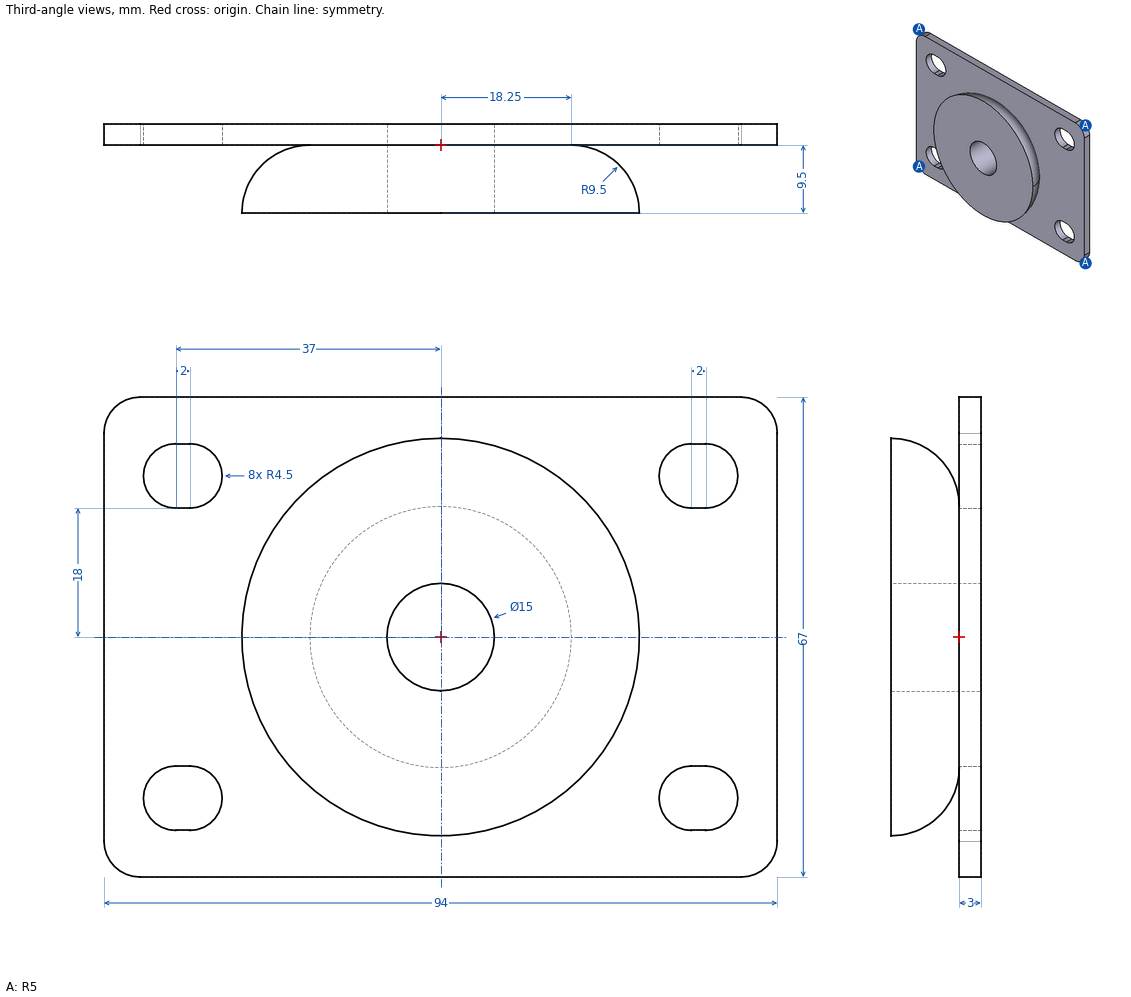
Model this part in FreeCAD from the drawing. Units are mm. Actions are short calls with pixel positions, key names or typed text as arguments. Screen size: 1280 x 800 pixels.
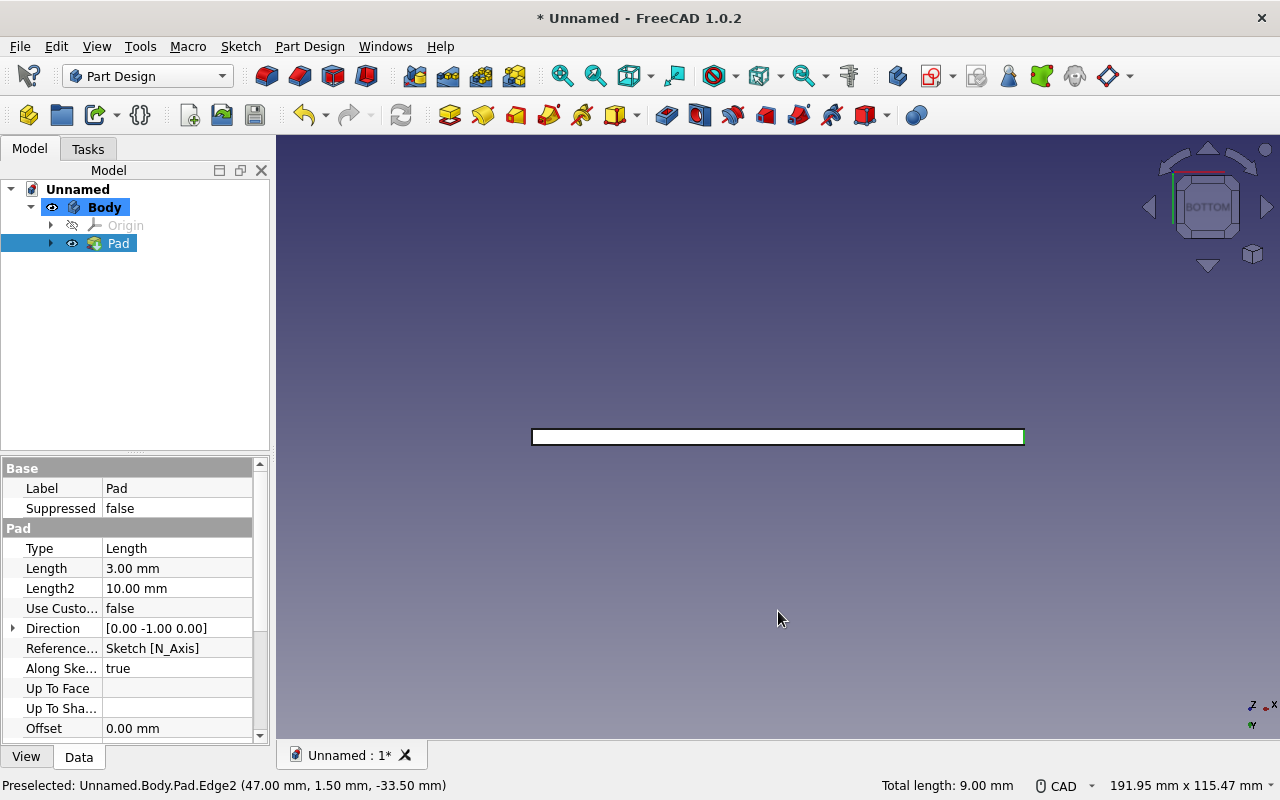
click(532, 436, ctrl)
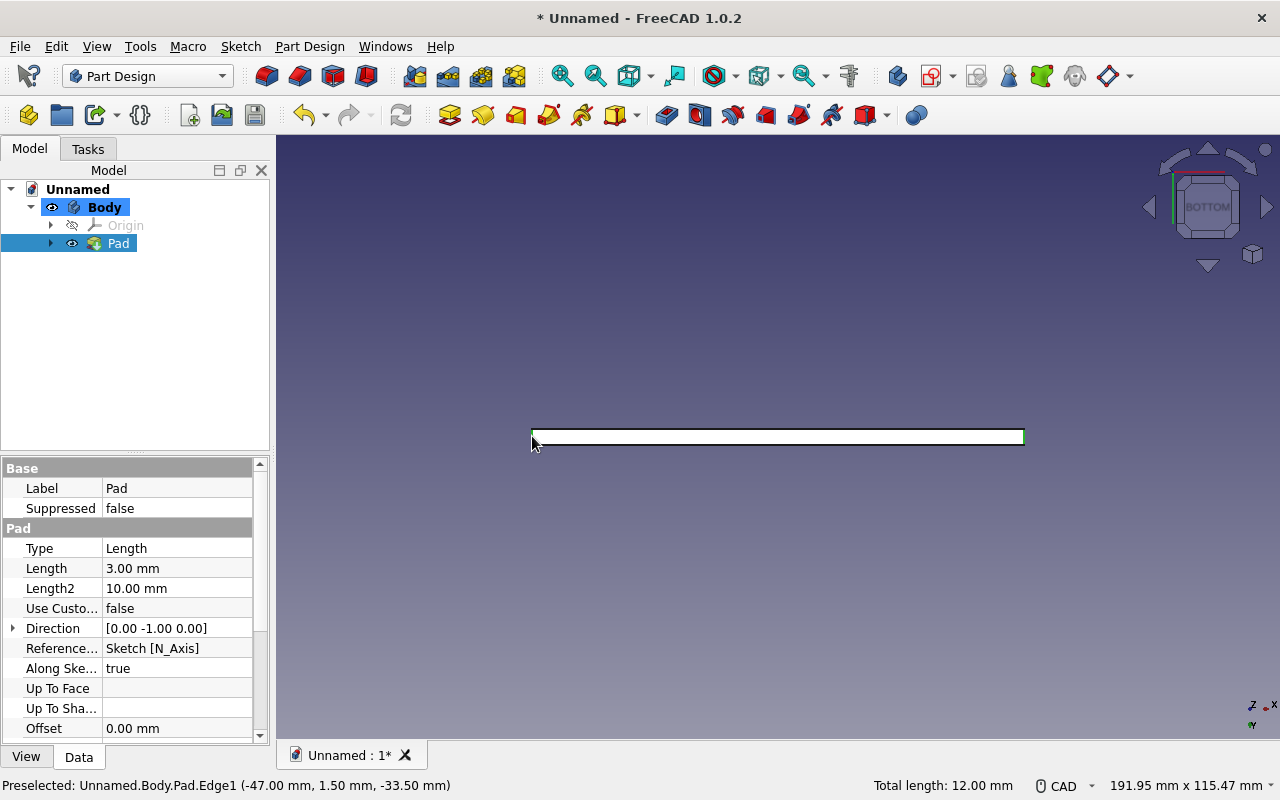
click(267, 76)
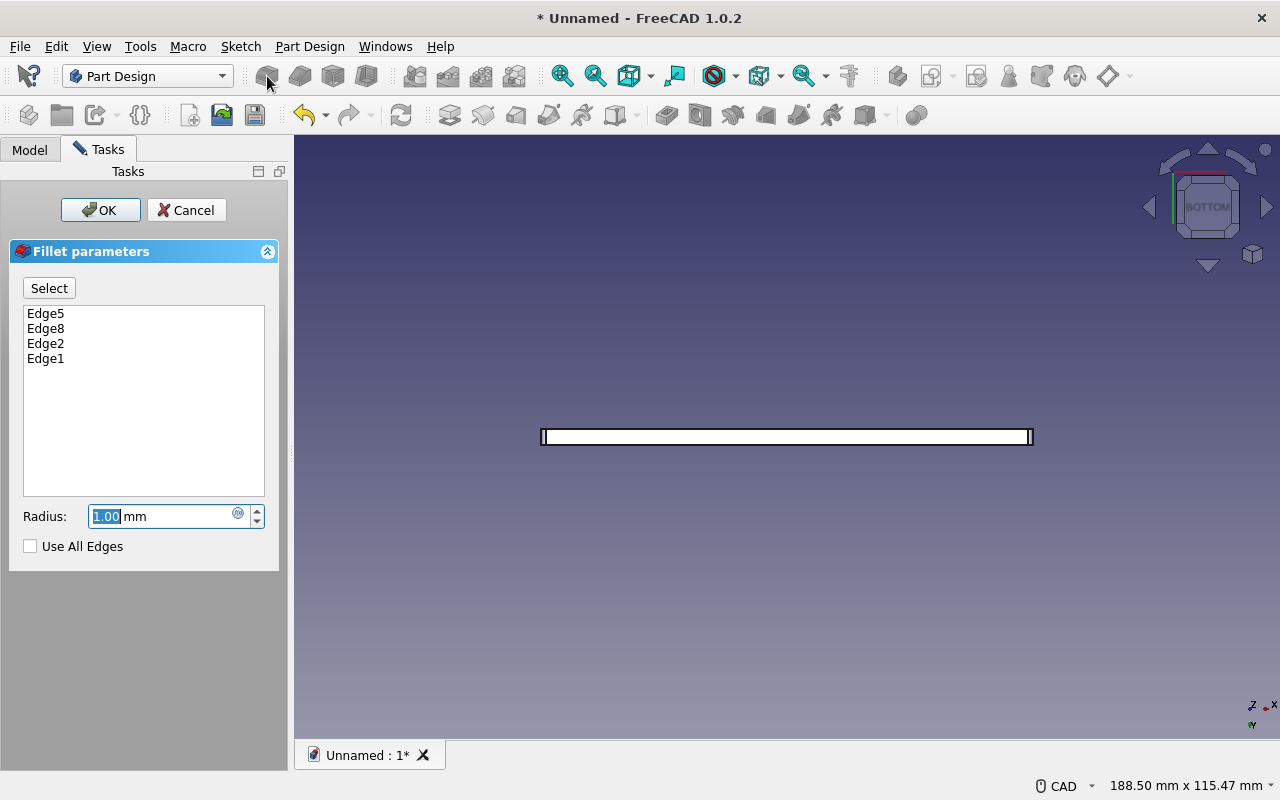
text(5)
key(Tab)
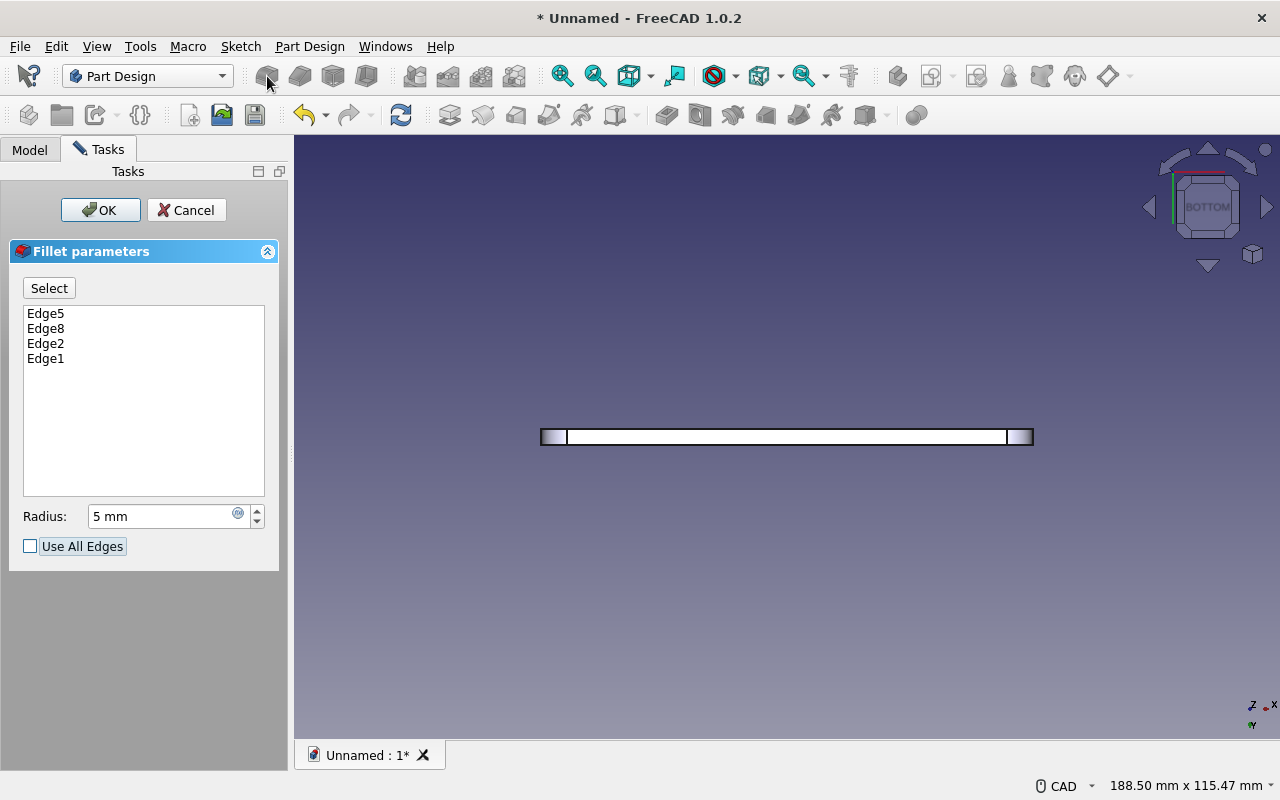
click(101, 210)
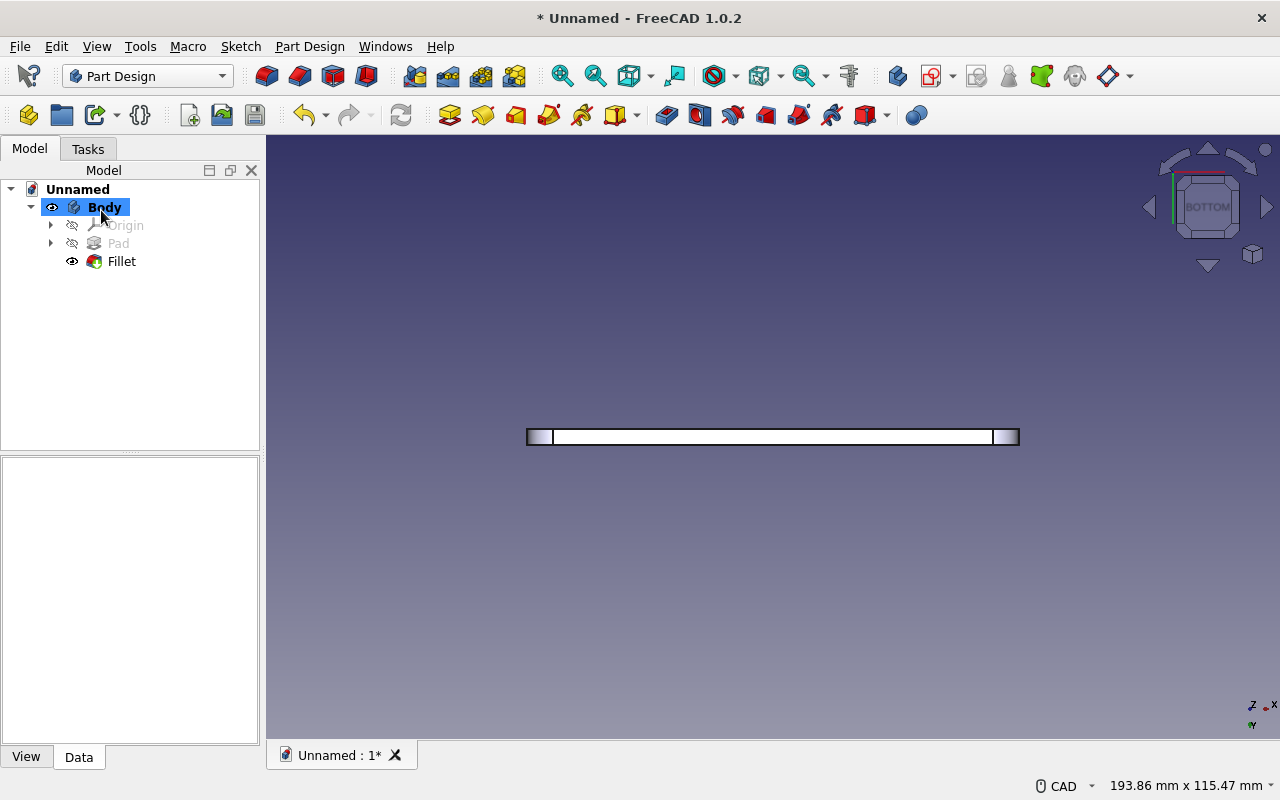
key(4)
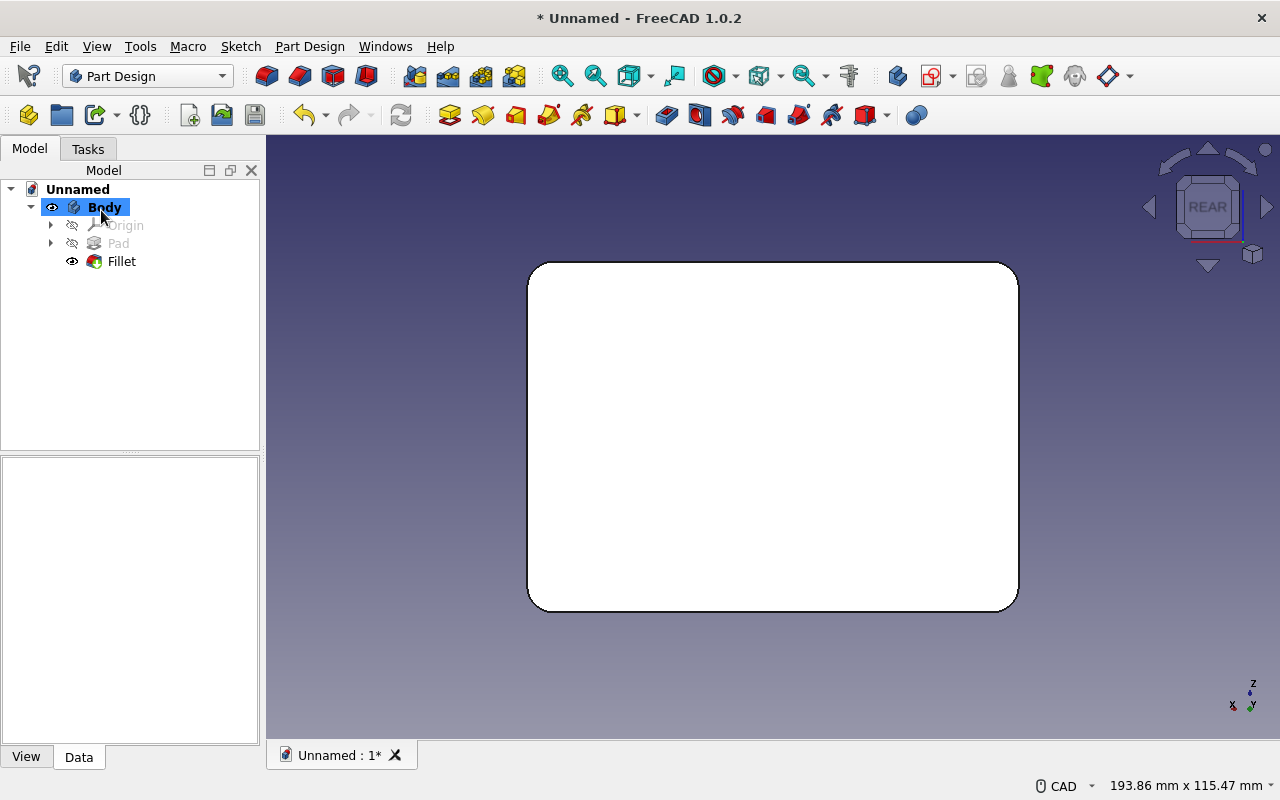
click(703, 436)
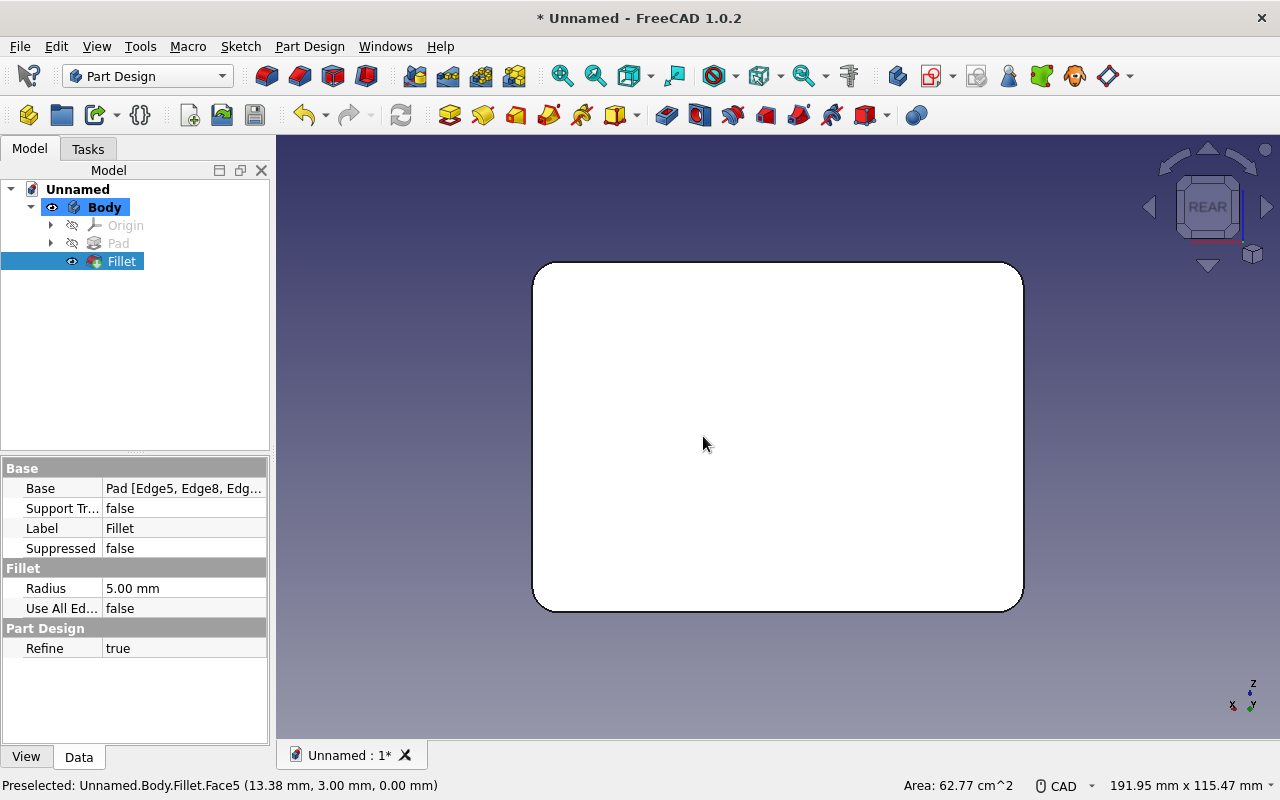
click(930, 76)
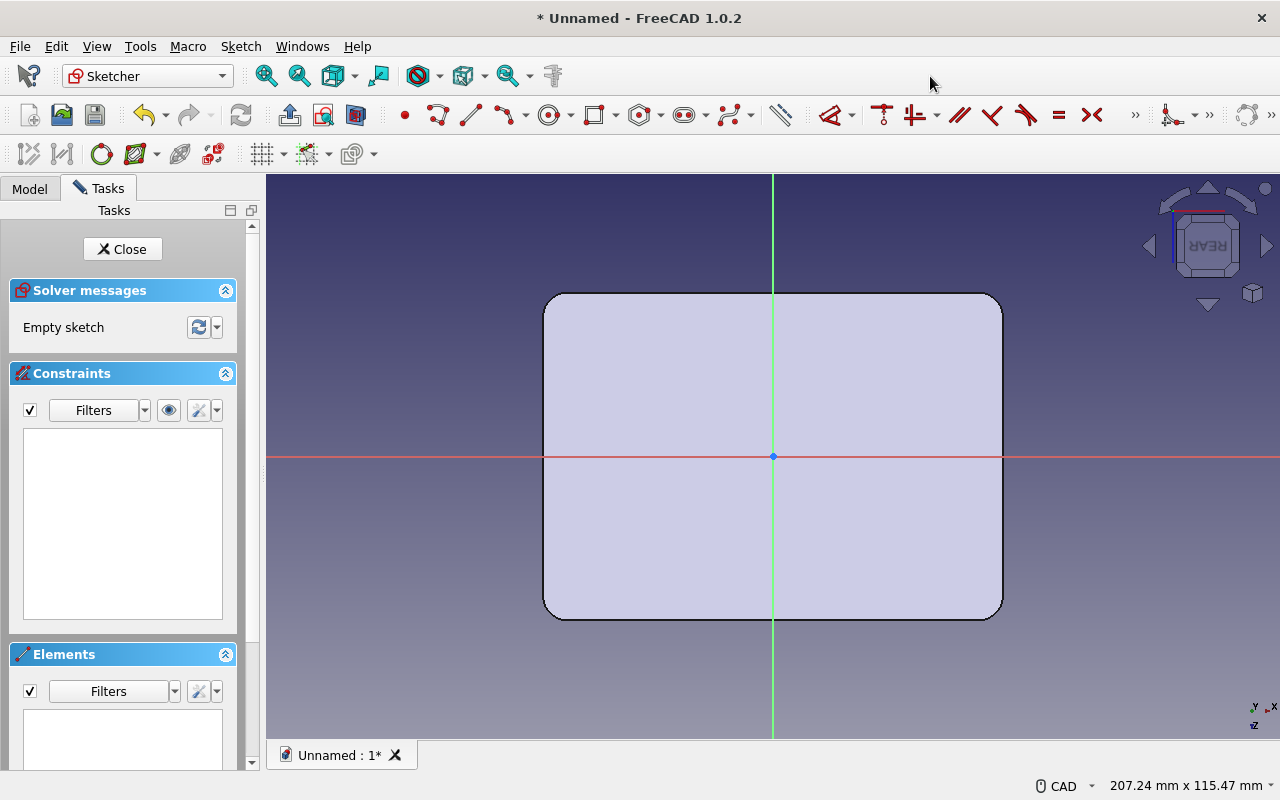
scroll(912, 457, up, 2)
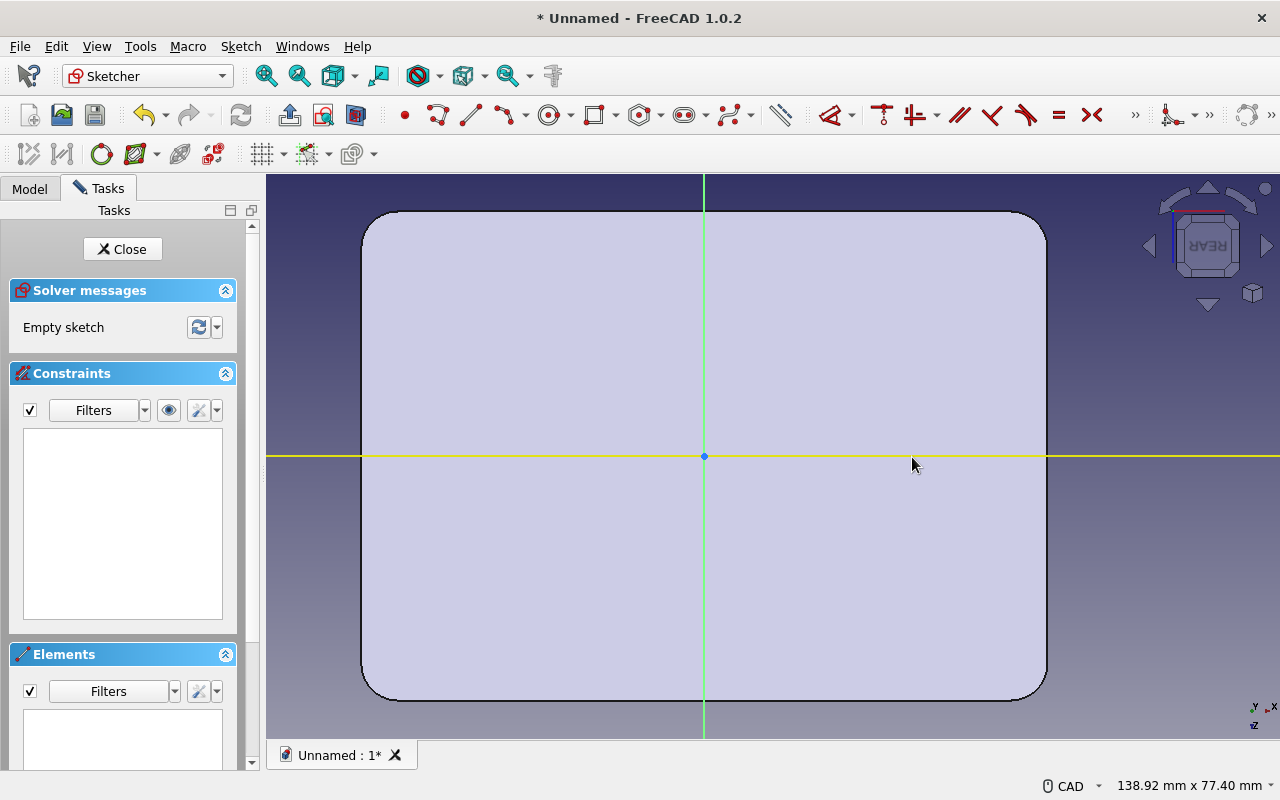
key(g)
key(s)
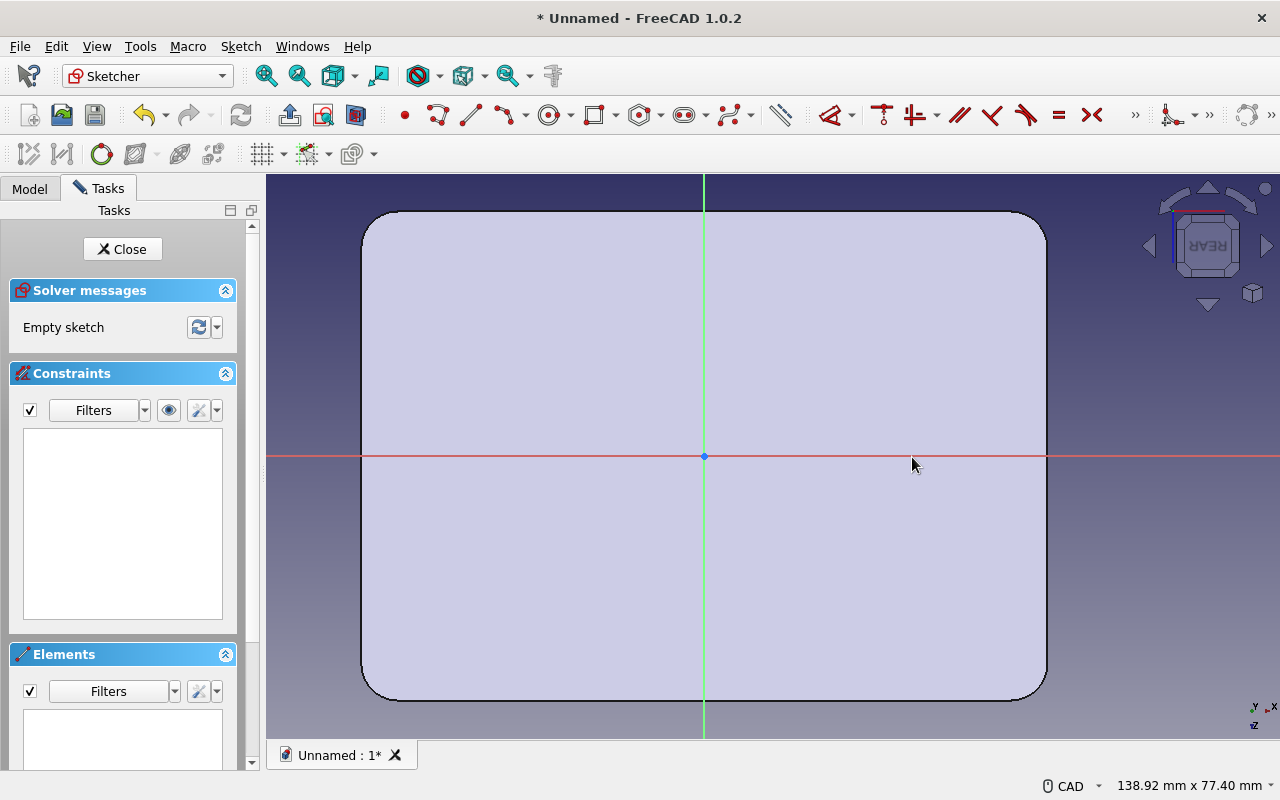
click(434, 620)